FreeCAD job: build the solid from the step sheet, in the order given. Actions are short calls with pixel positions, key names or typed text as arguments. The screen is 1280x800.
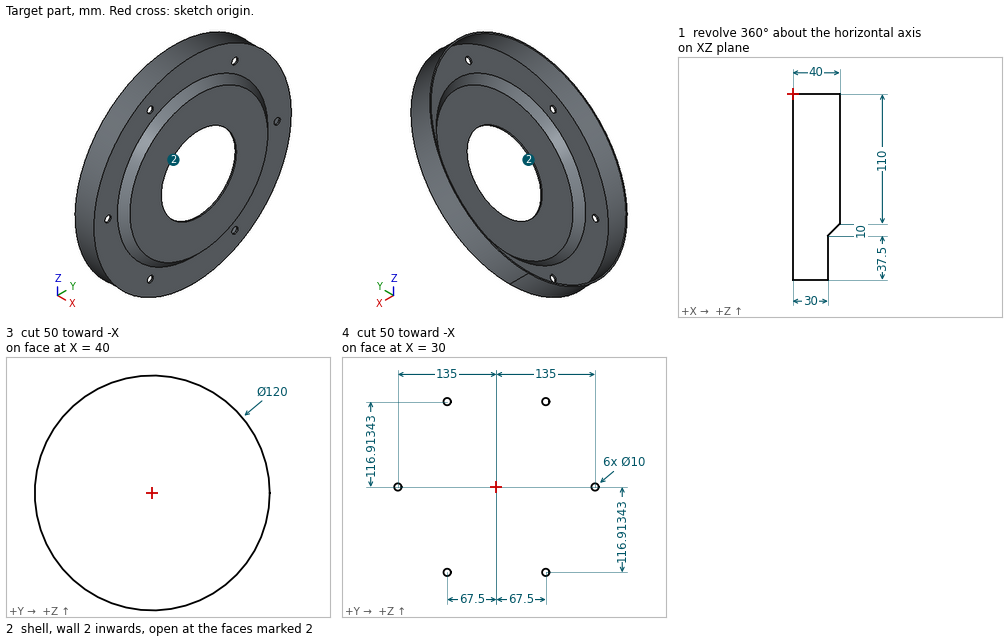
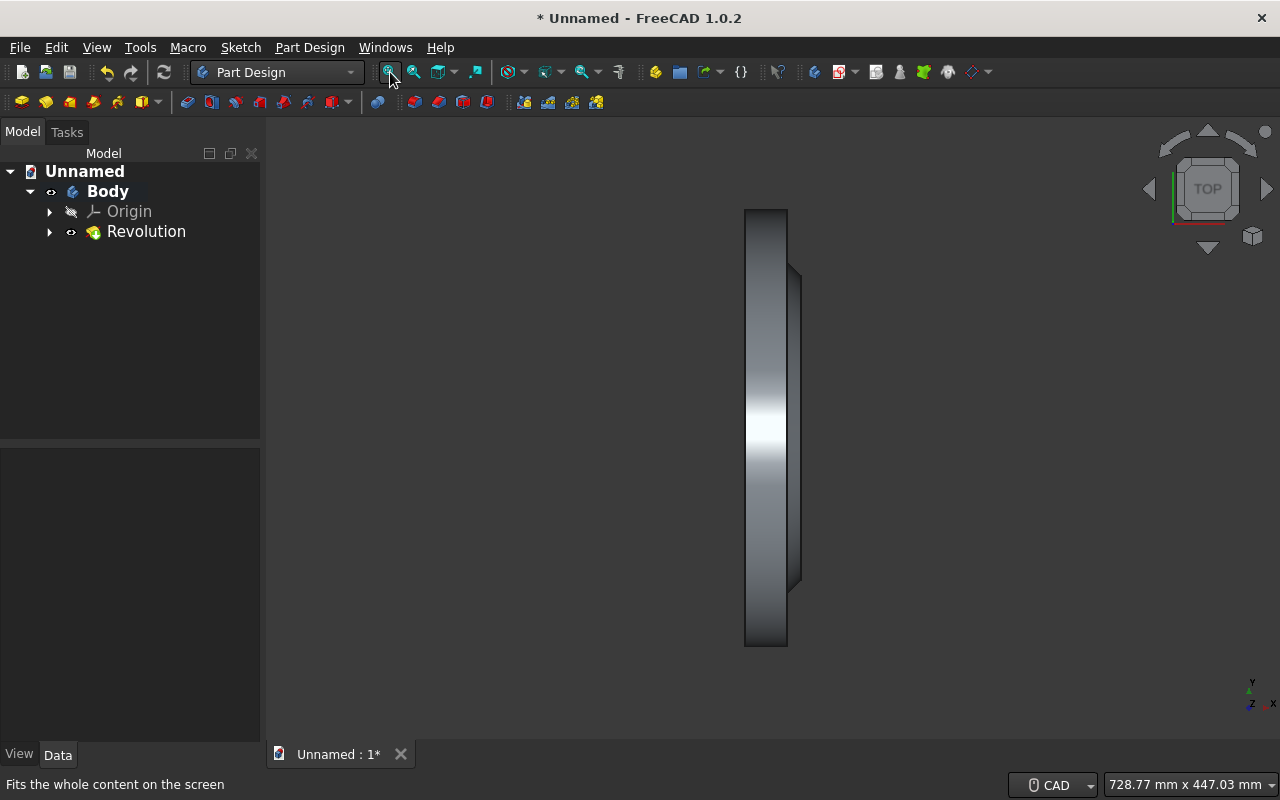
key(1)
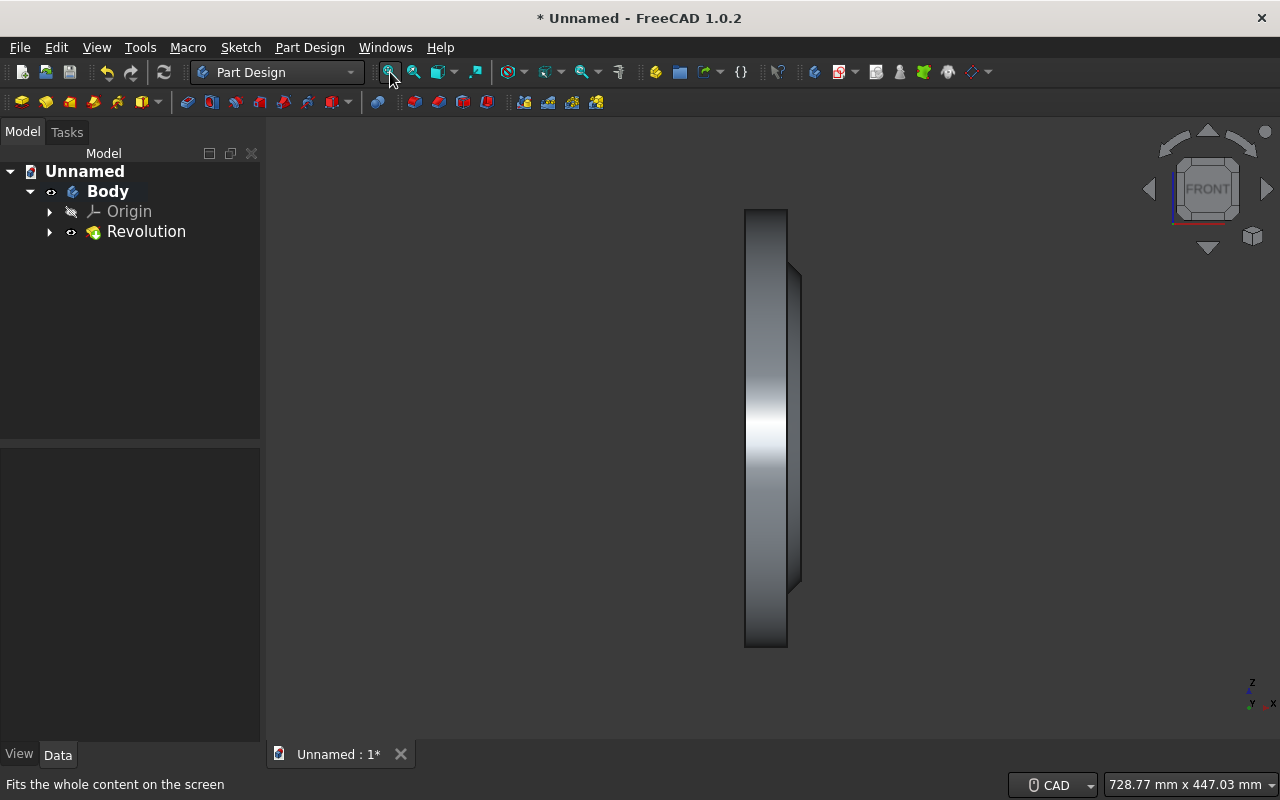
key(3)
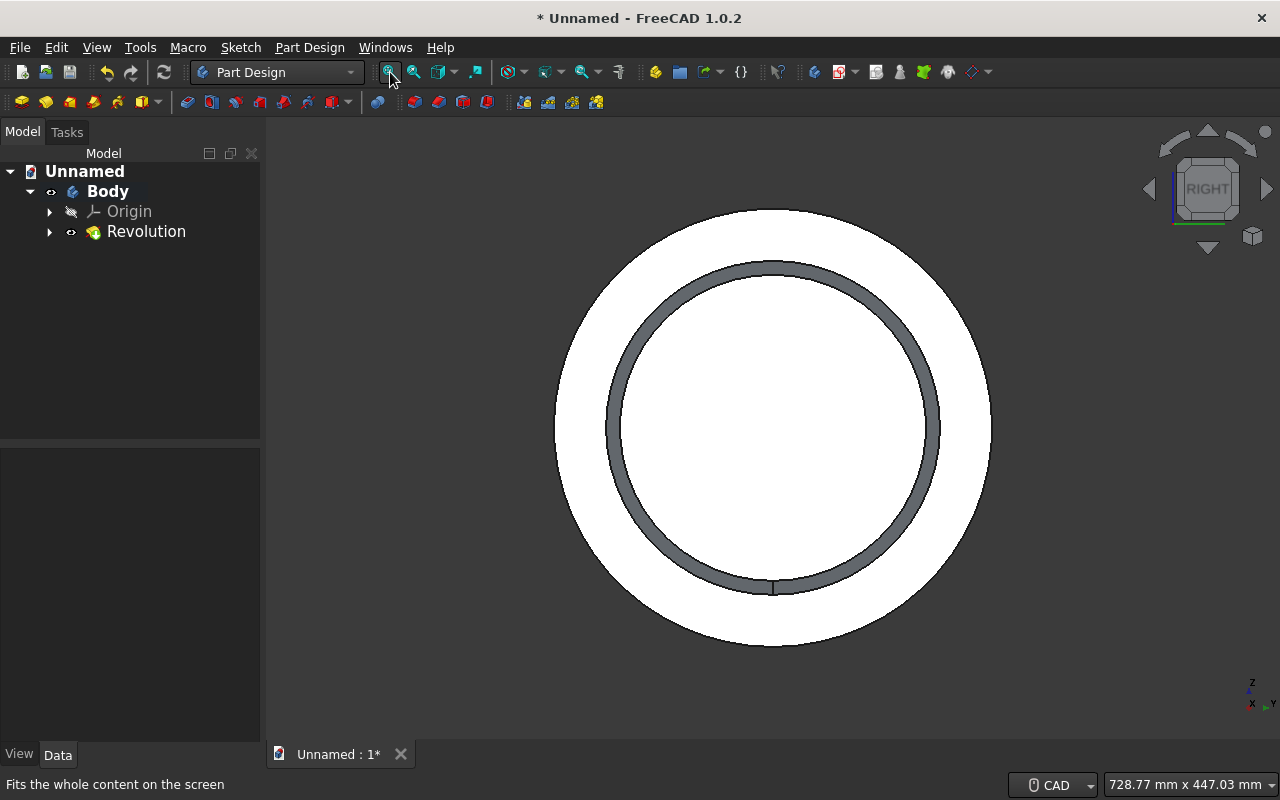
key(5)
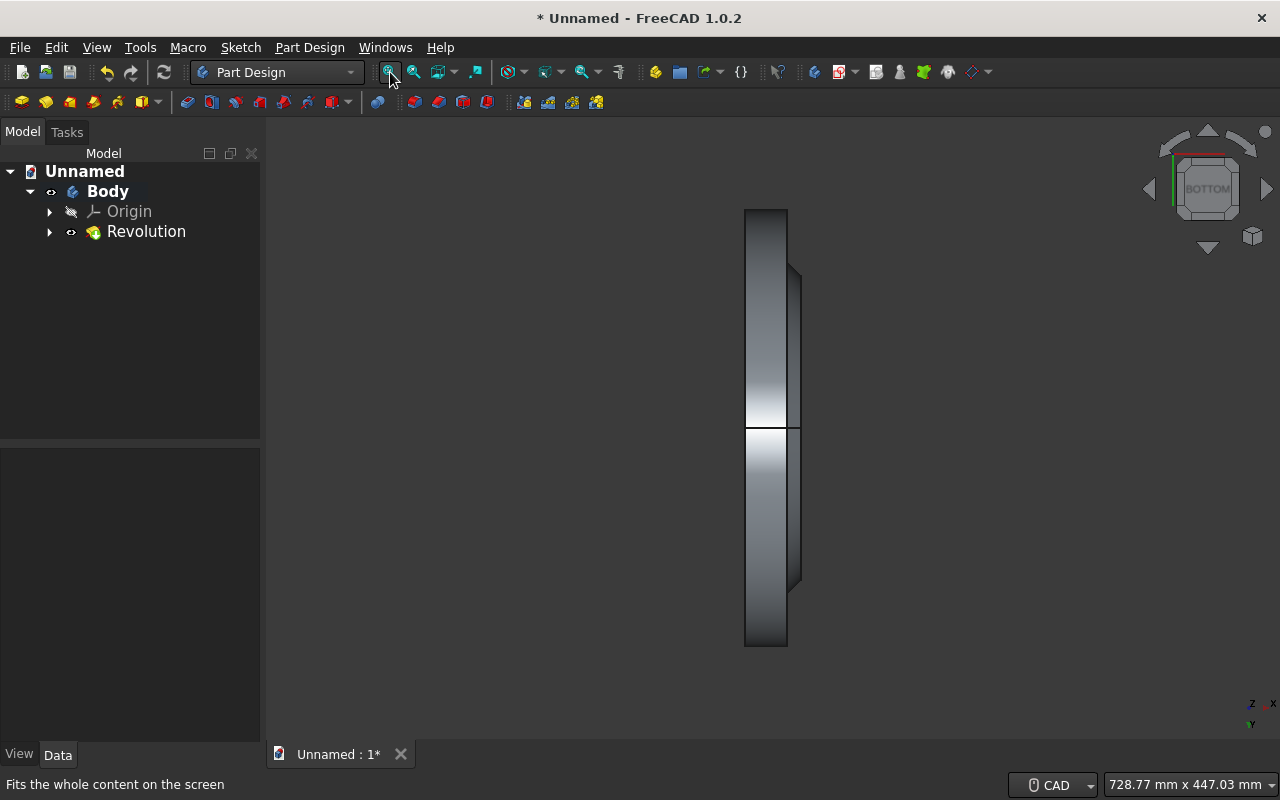
key(4)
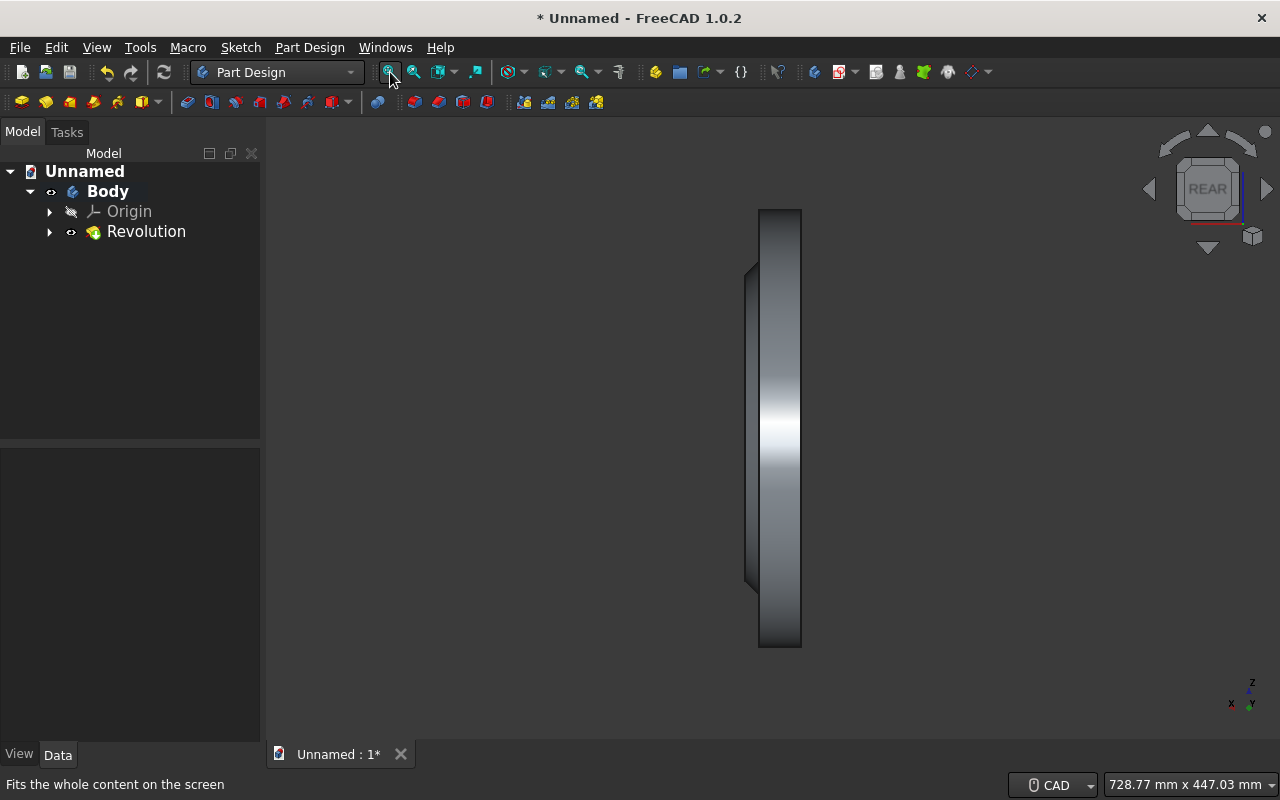
key(6)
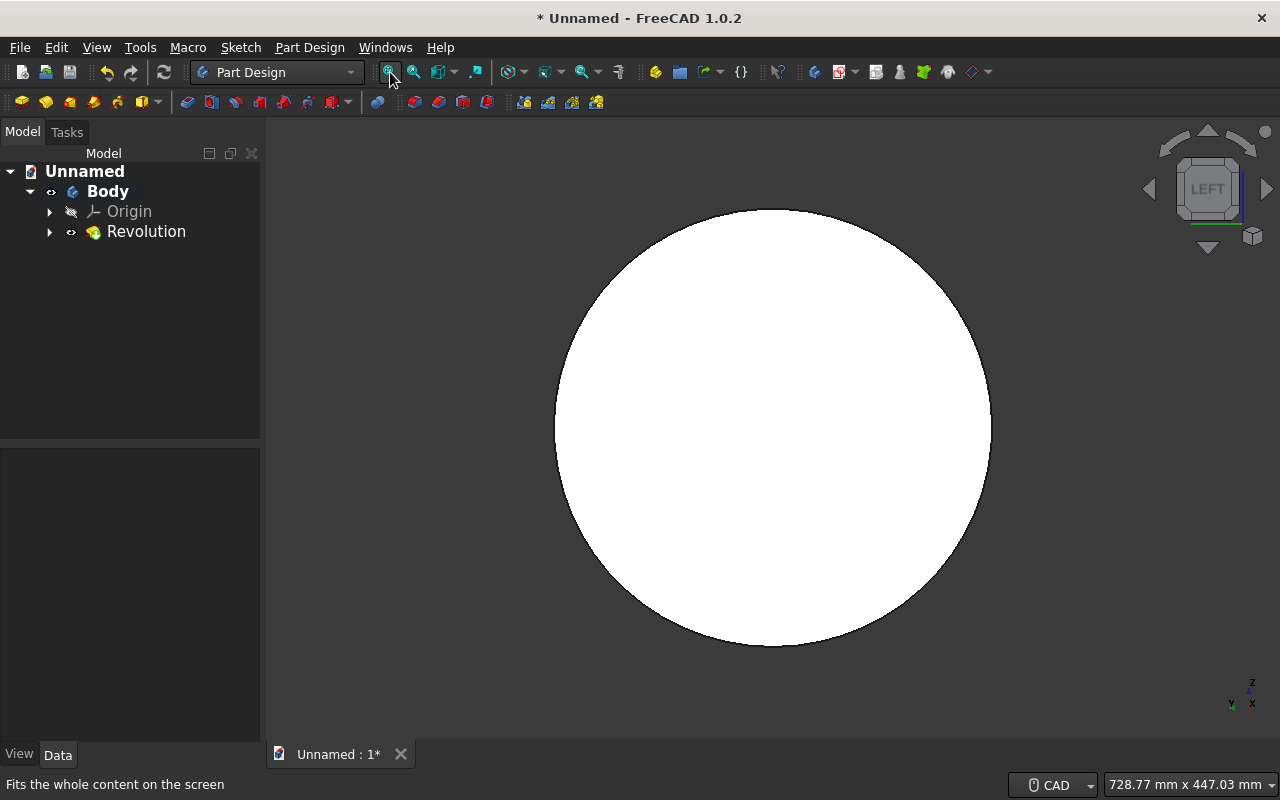
click(773, 427)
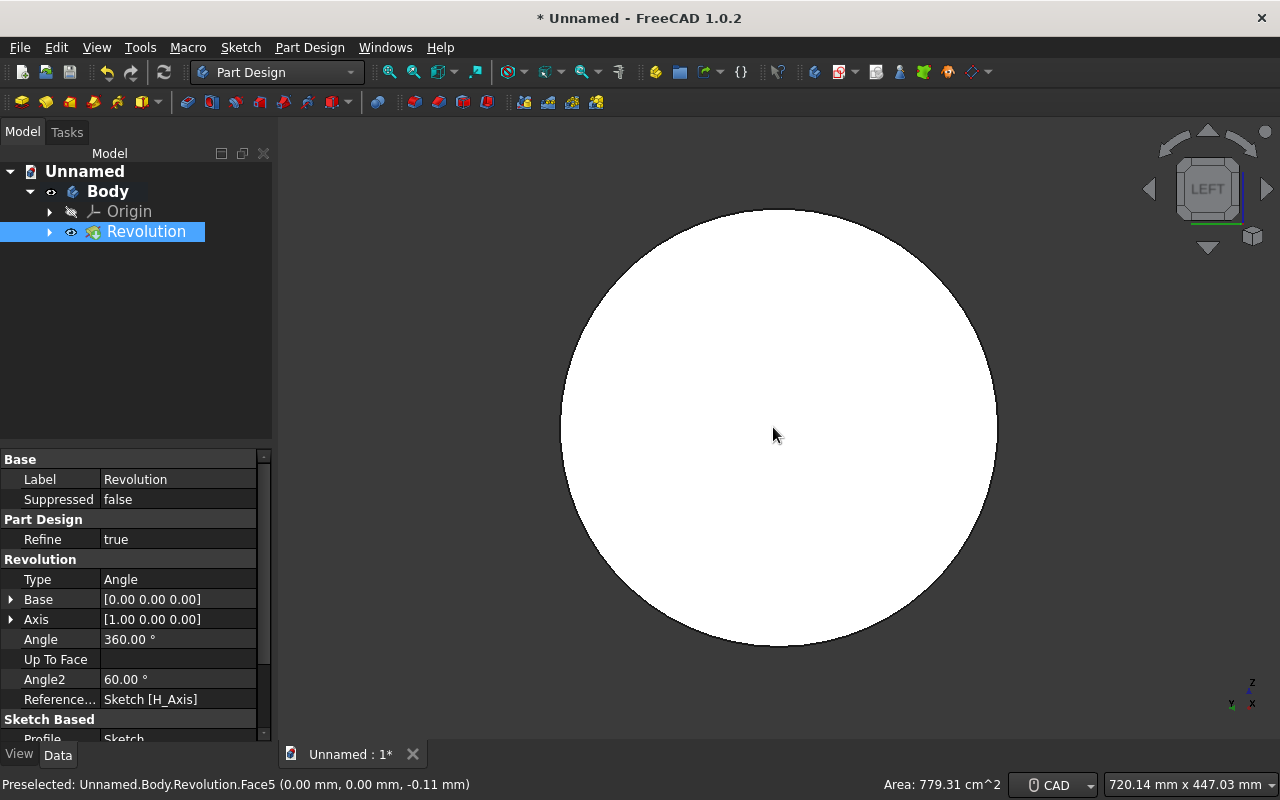
click(488, 102)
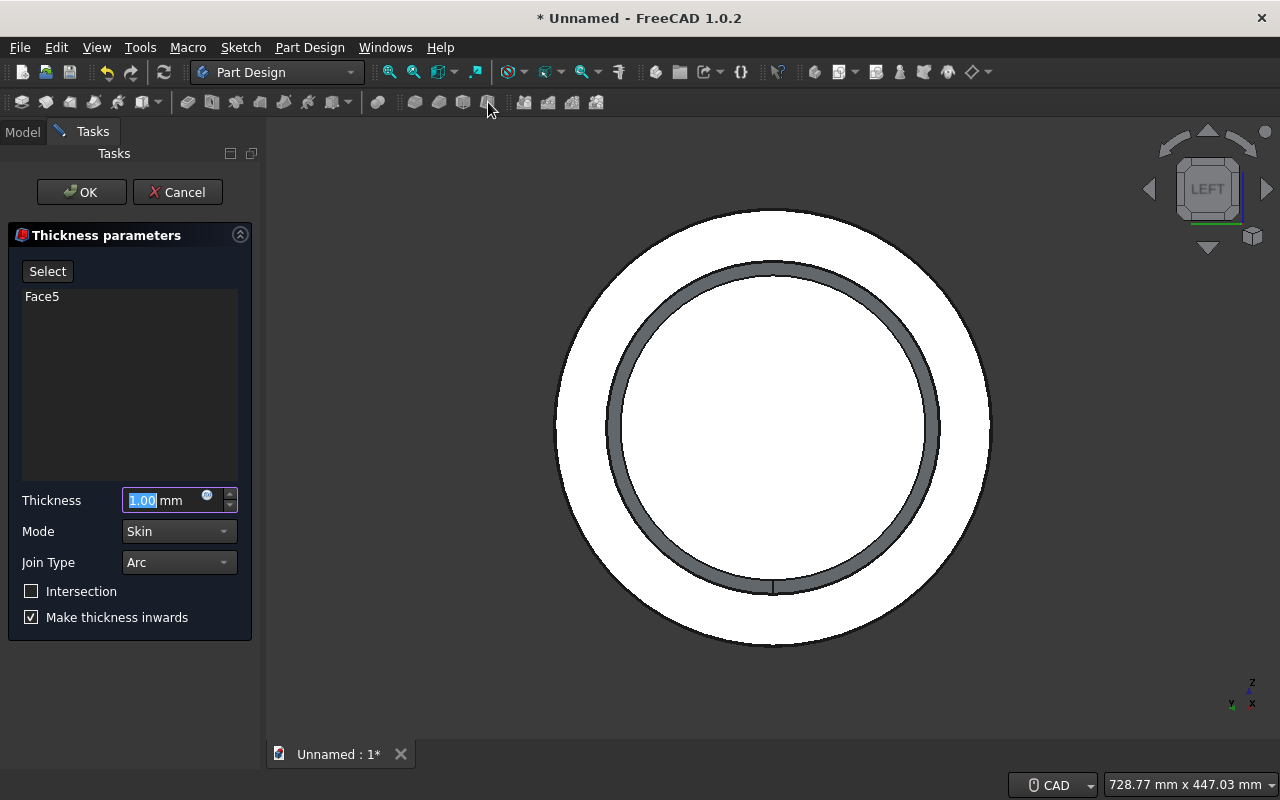
text(2)
key(Tab)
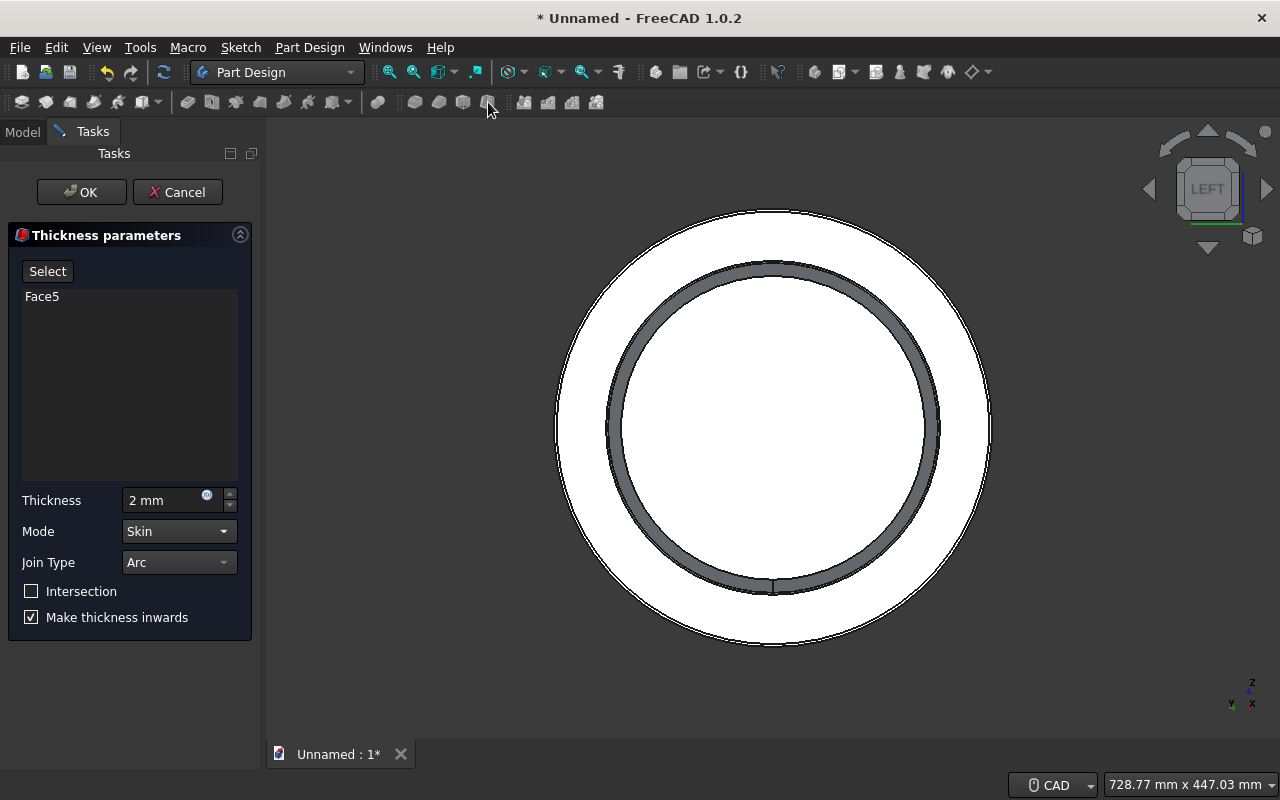
click(180, 562)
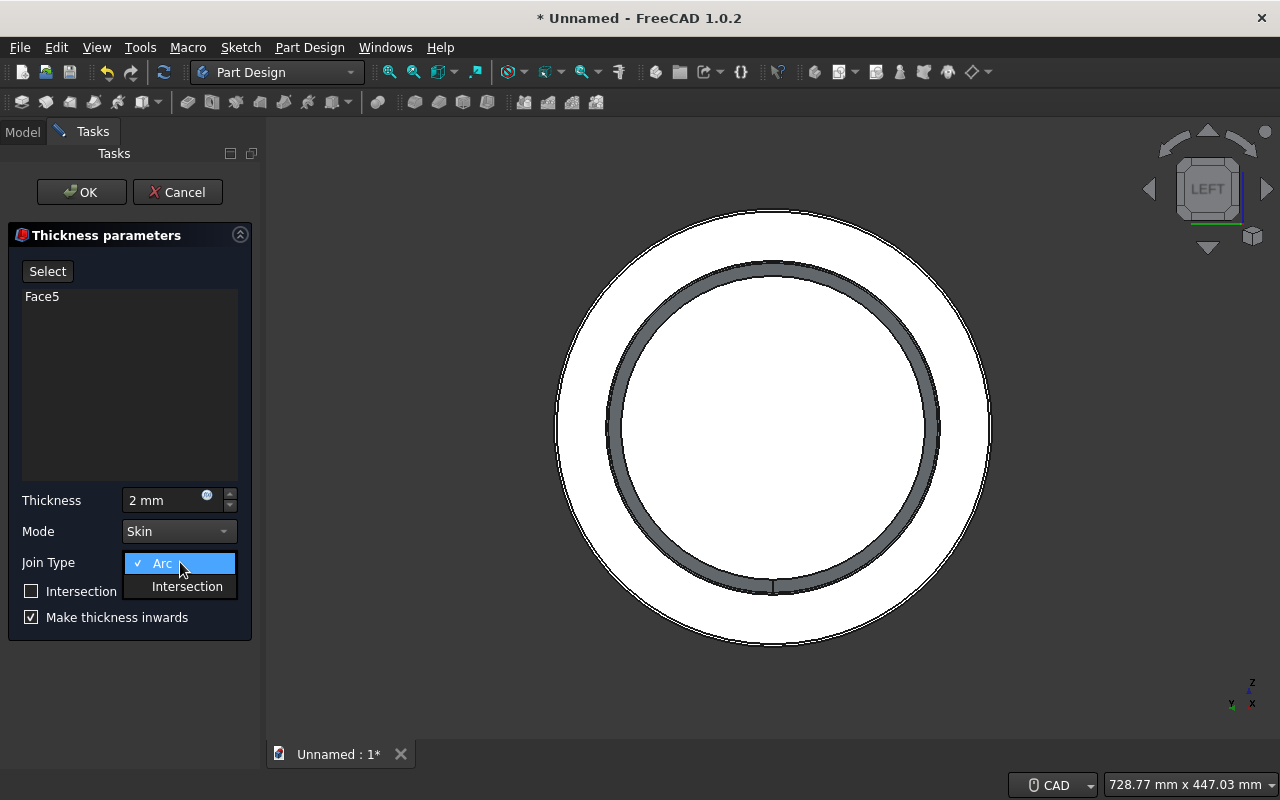
click(179, 586)